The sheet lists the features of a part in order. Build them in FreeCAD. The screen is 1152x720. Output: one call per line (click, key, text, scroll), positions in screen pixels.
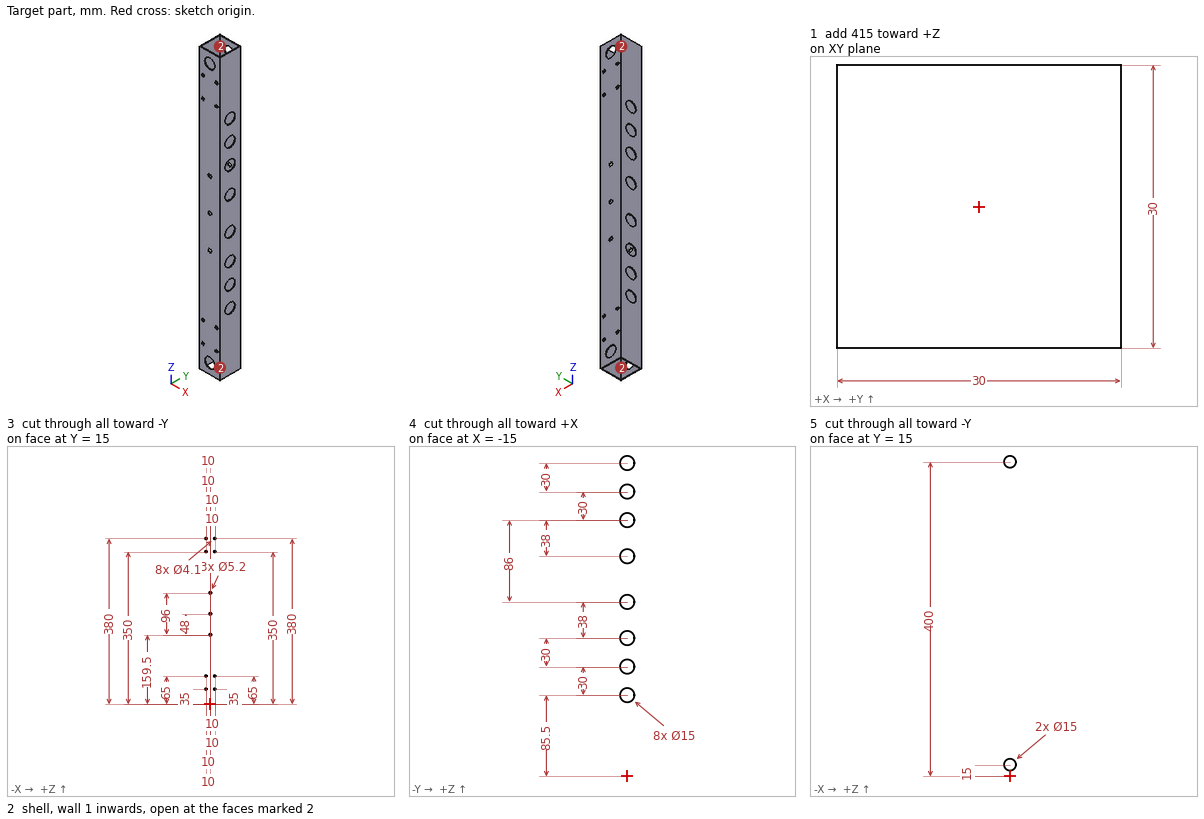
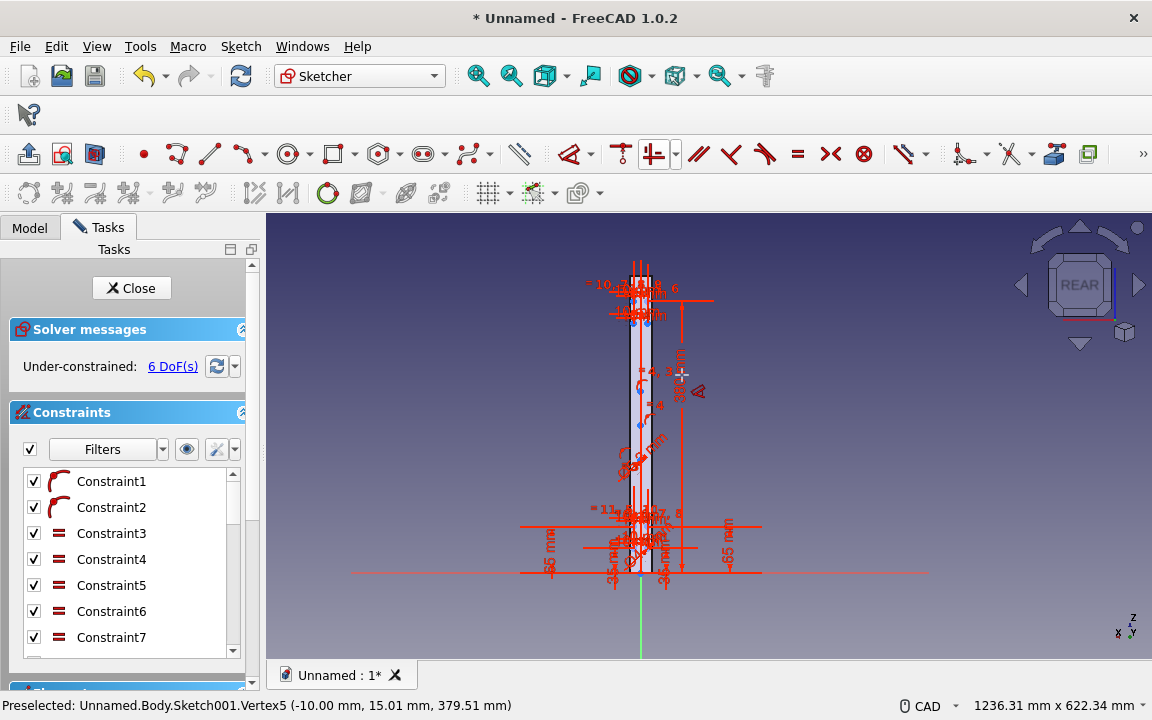
click(648, 323)
click(607, 391)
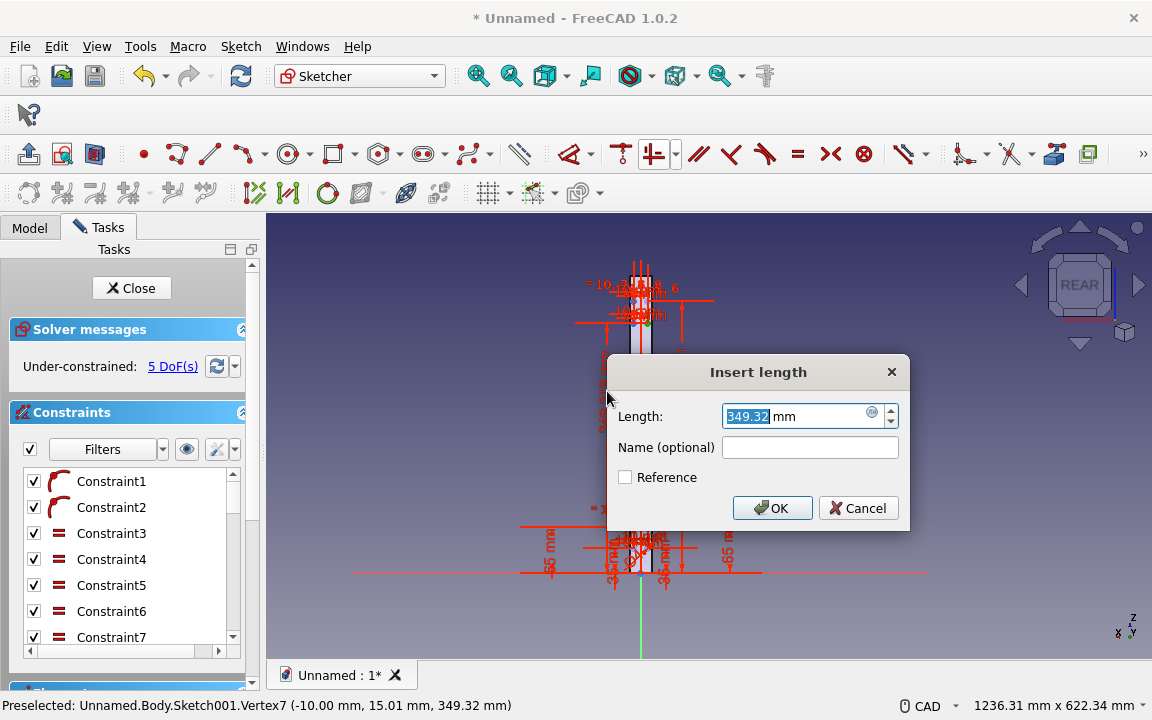
text(350)
key(Return)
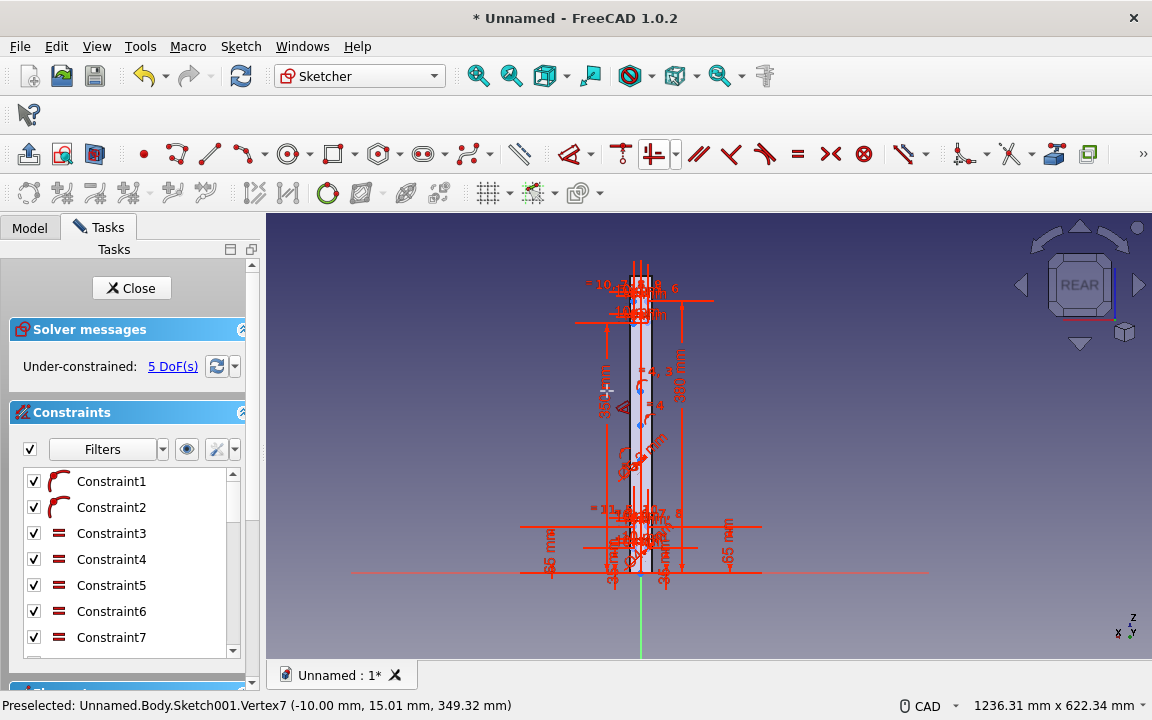
click(634, 323)
click(600, 361)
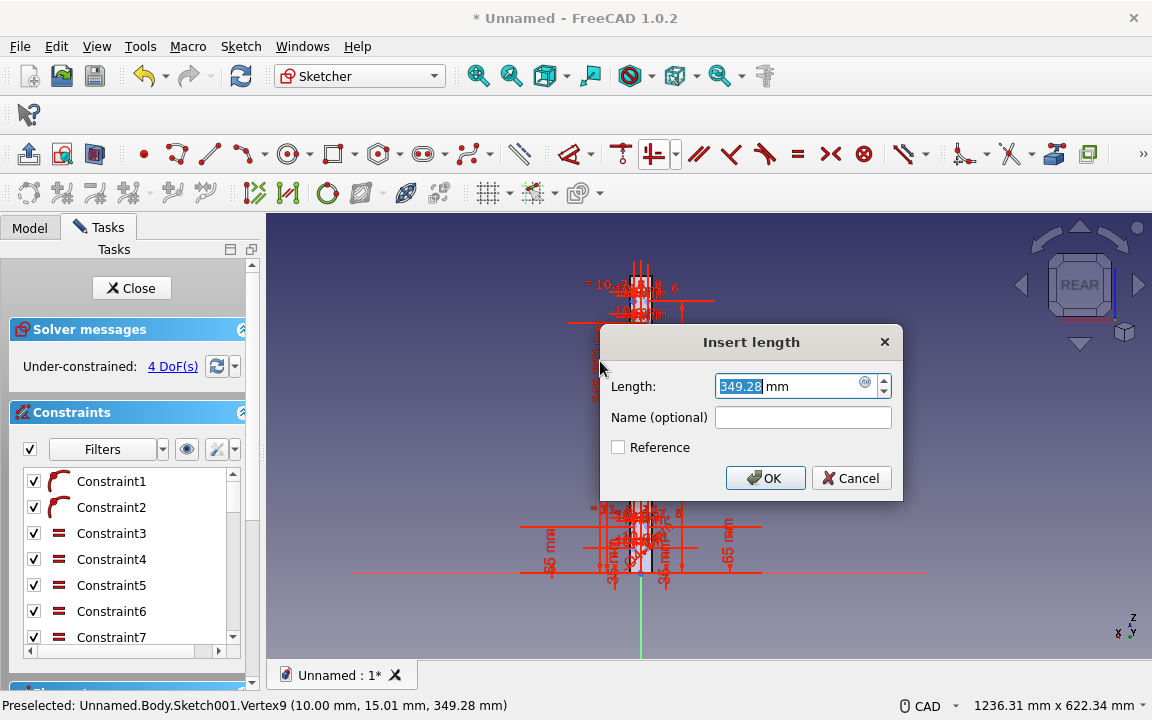
text(350)
key(Return)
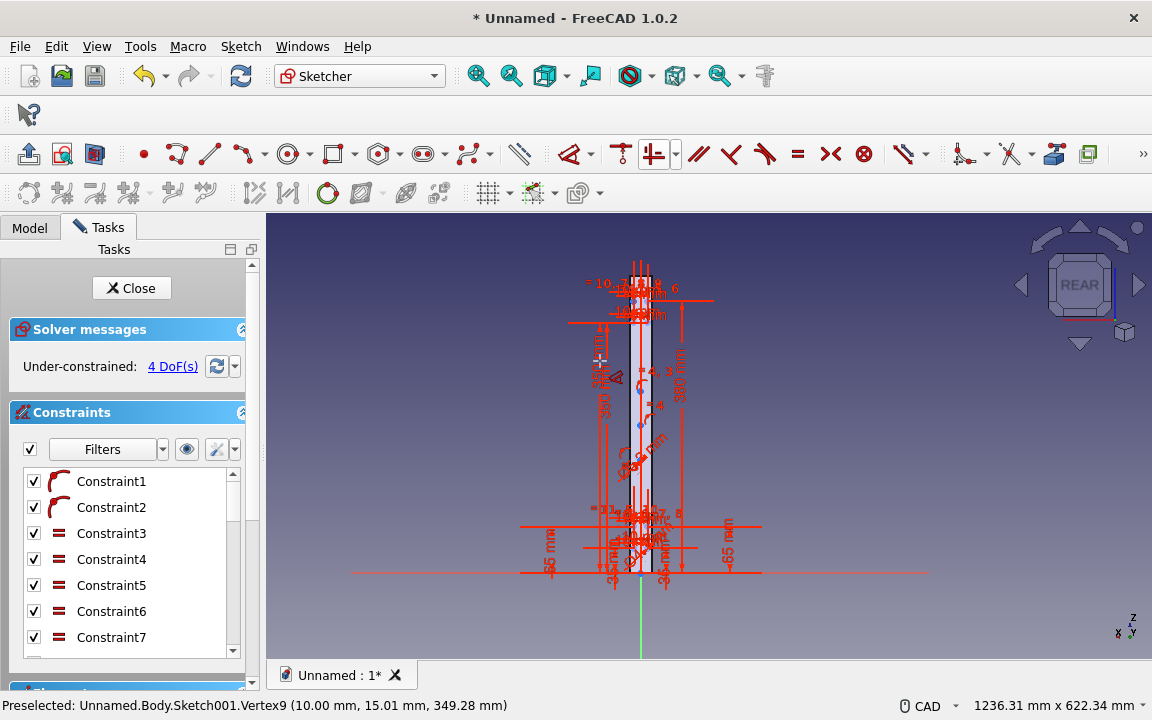
click(634, 302)
click(675, 342)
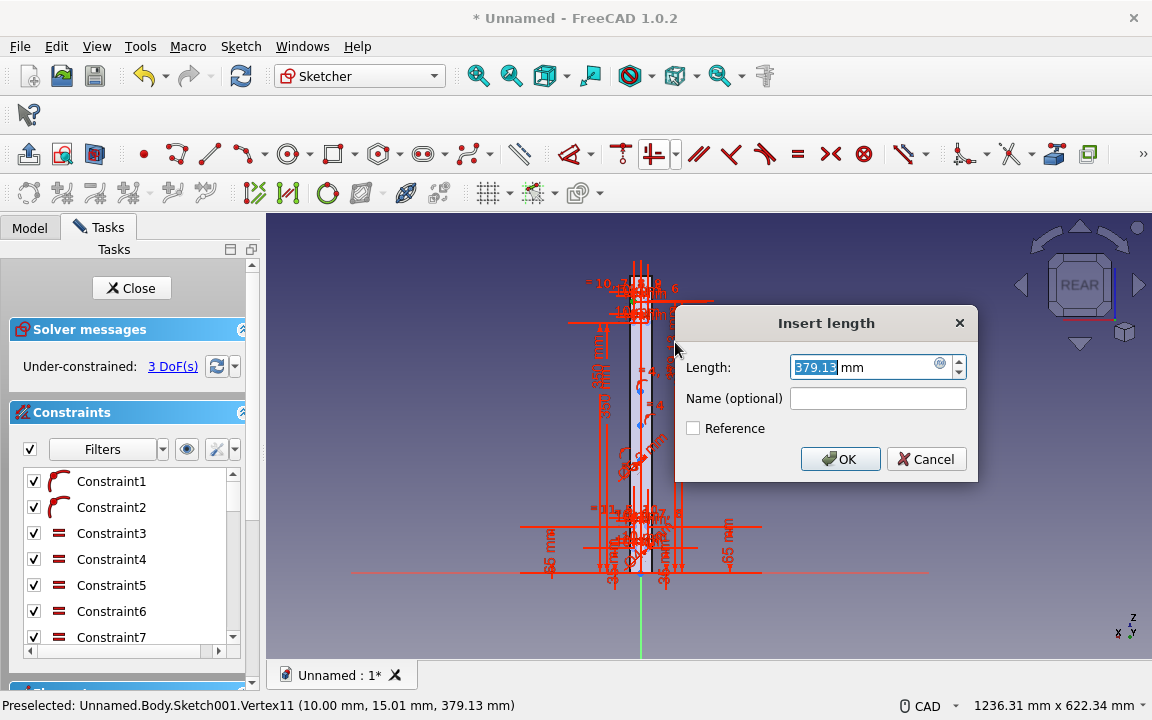
text(380)
key(Return)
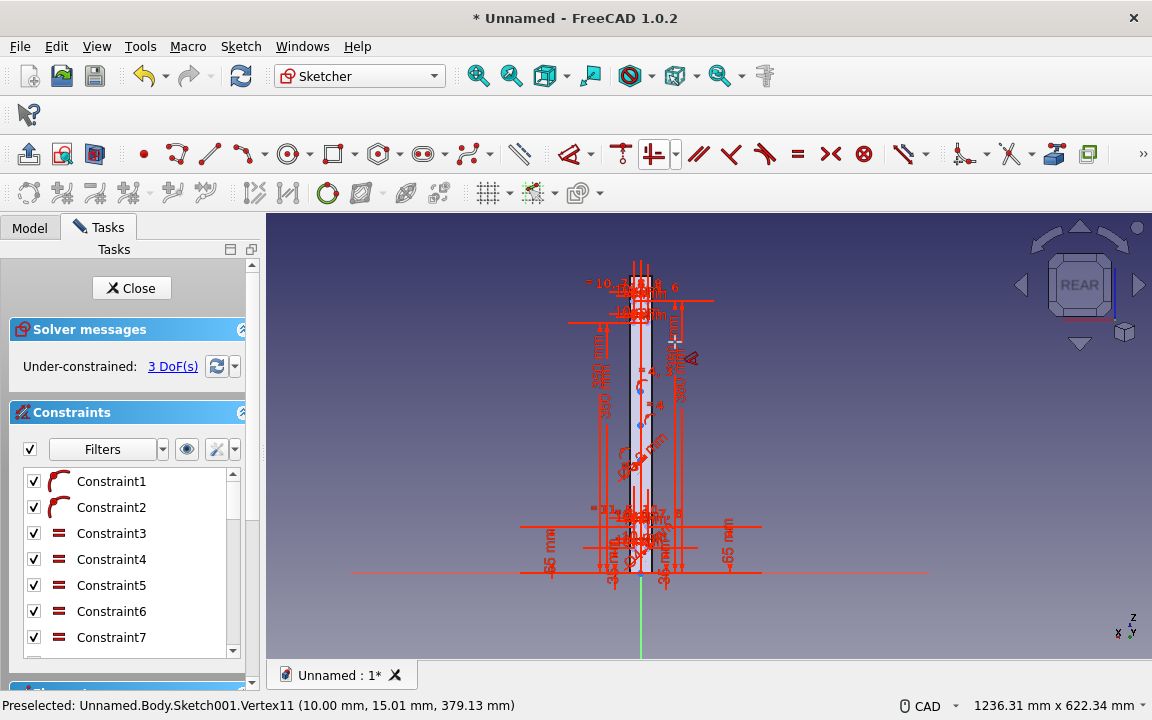
click(641, 460)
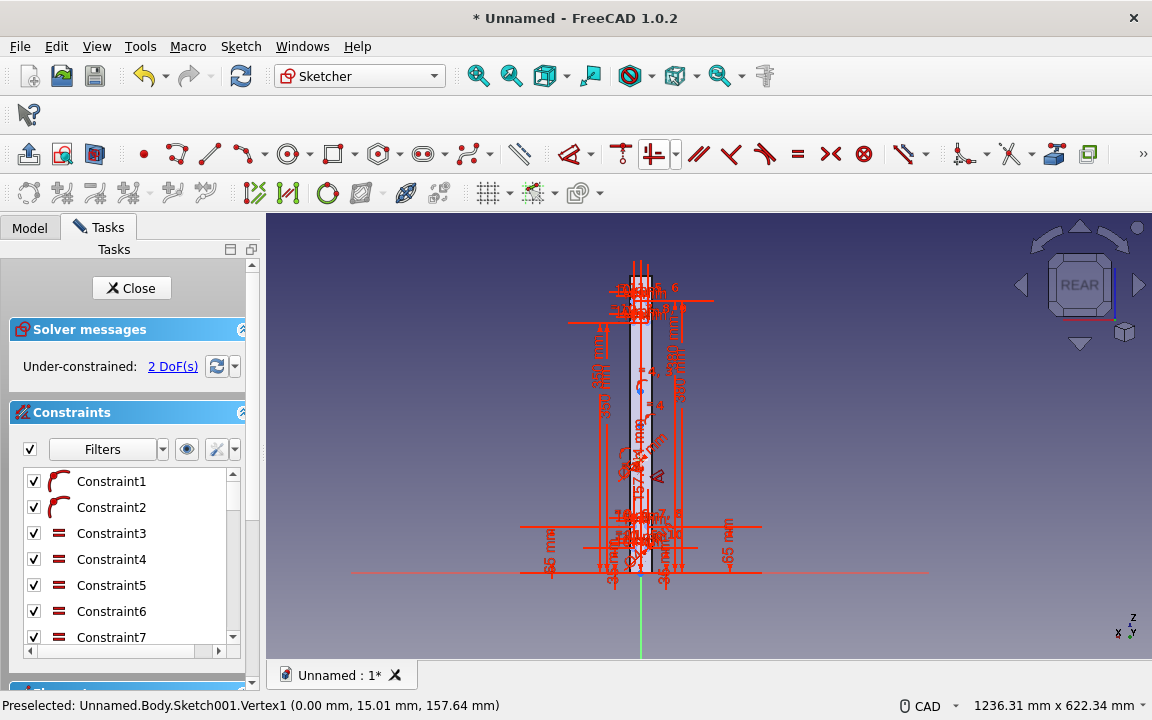
click(641, 391)
click(675, 426)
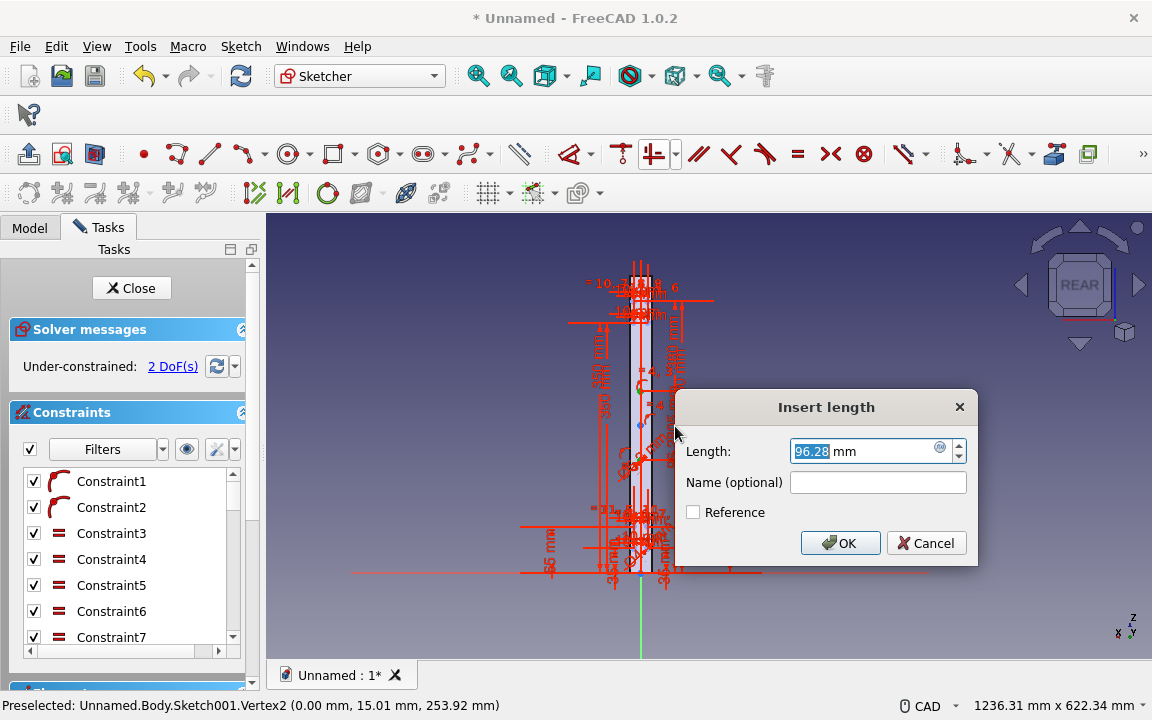
text(96)
key(Return)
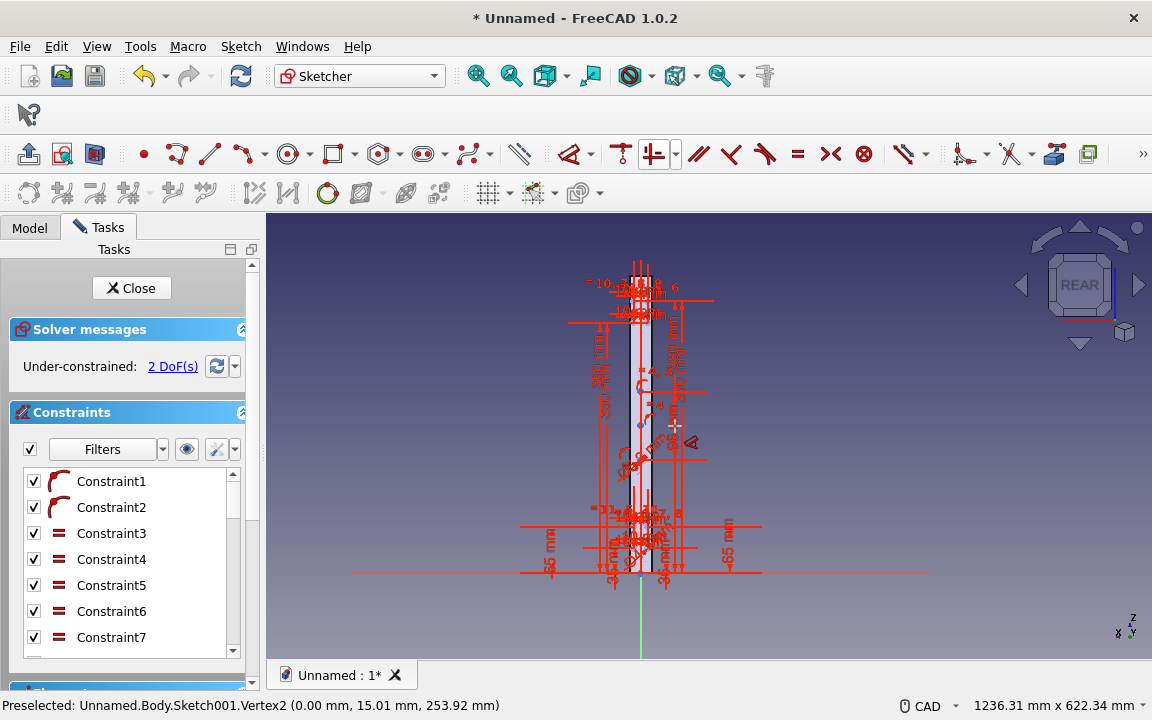
click(641, 460)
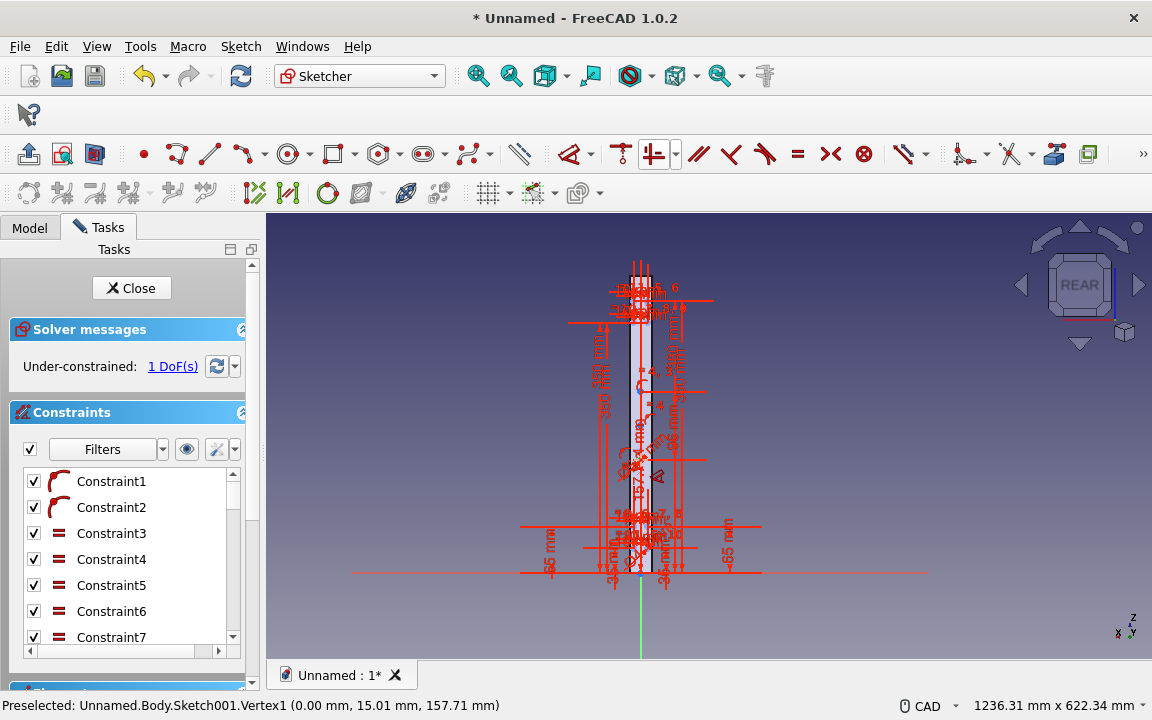
click(641, 425)
click(583, 435)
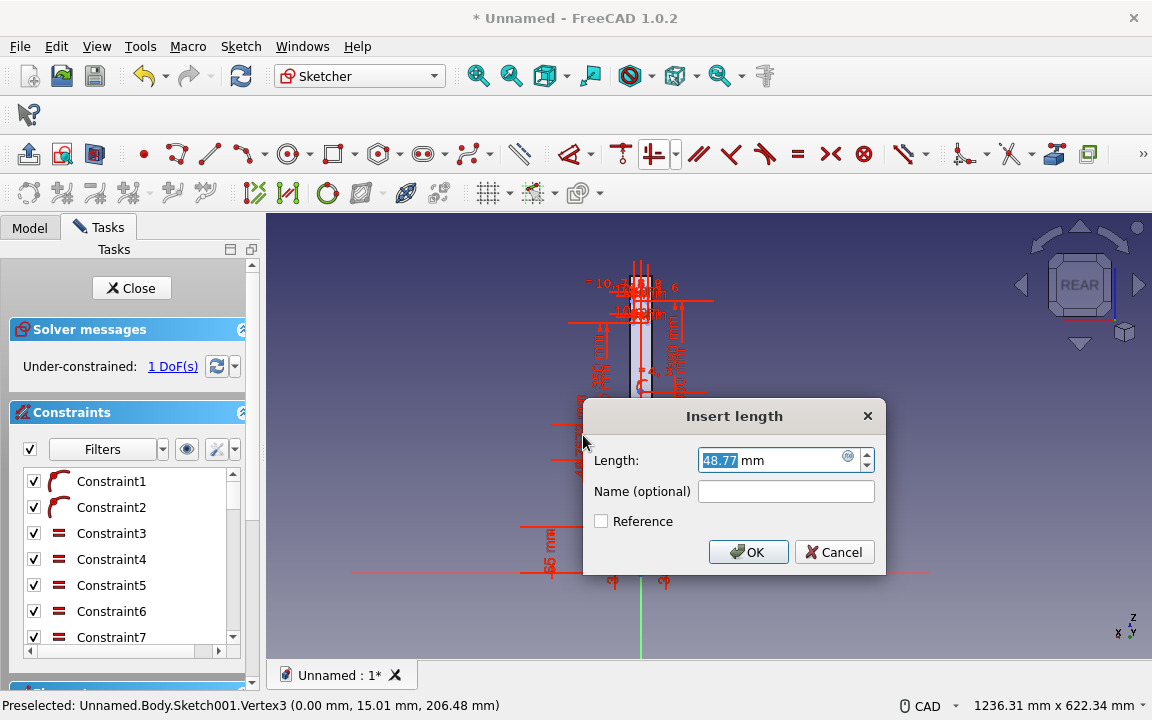
text(48)
key(Return)